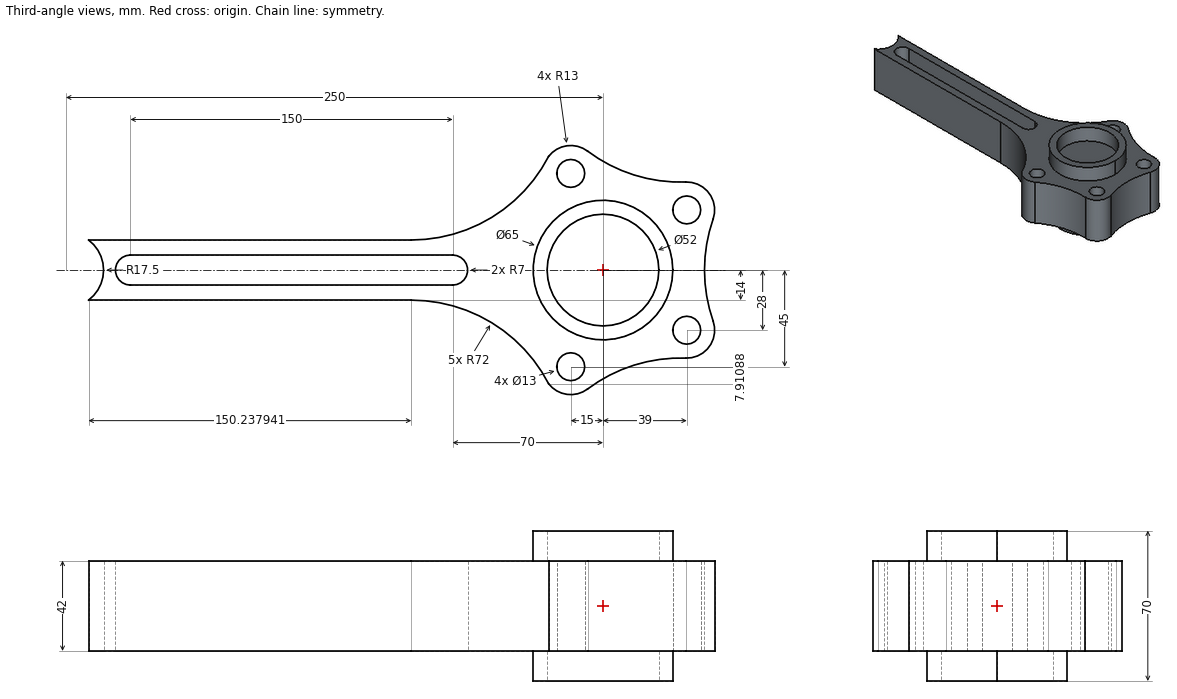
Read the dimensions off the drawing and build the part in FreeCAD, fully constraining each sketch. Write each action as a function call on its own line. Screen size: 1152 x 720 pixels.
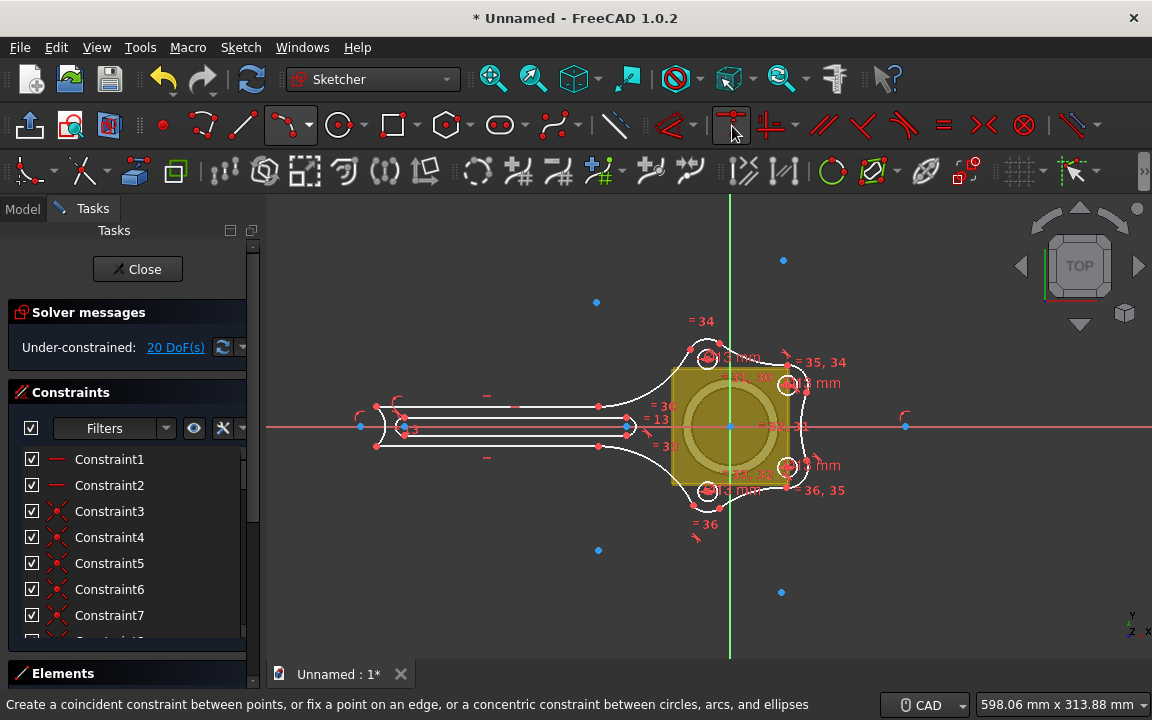
click(784, 261)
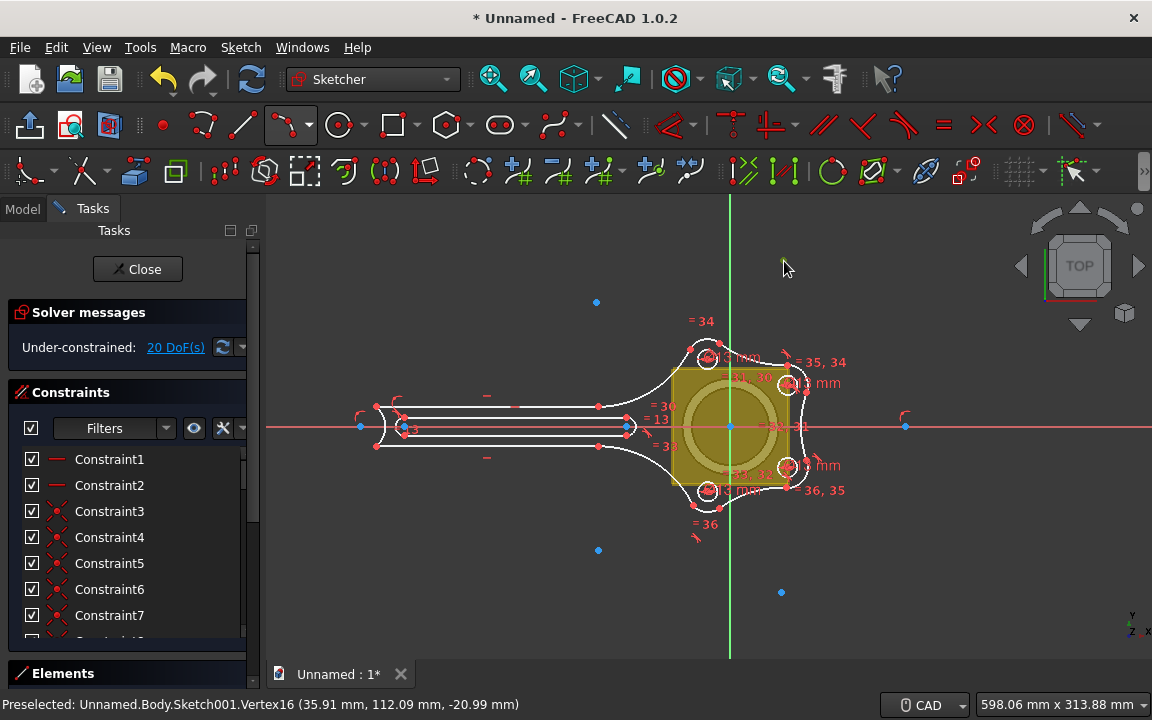
click(782, 592)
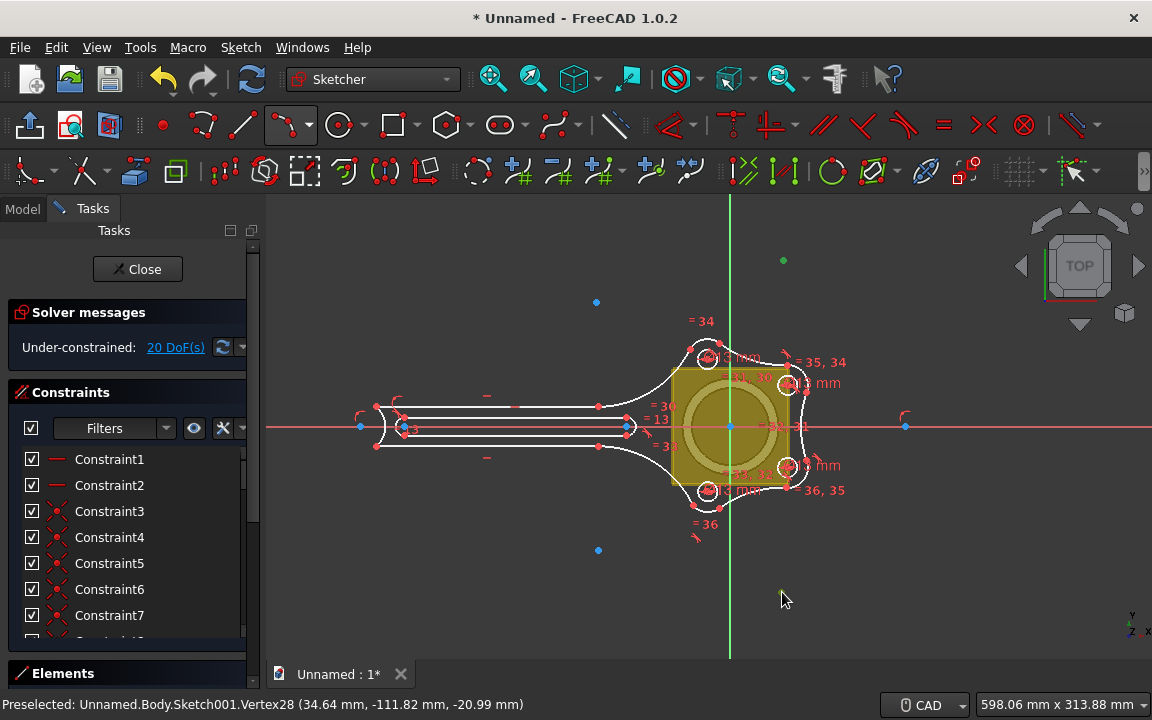
click(343, 427)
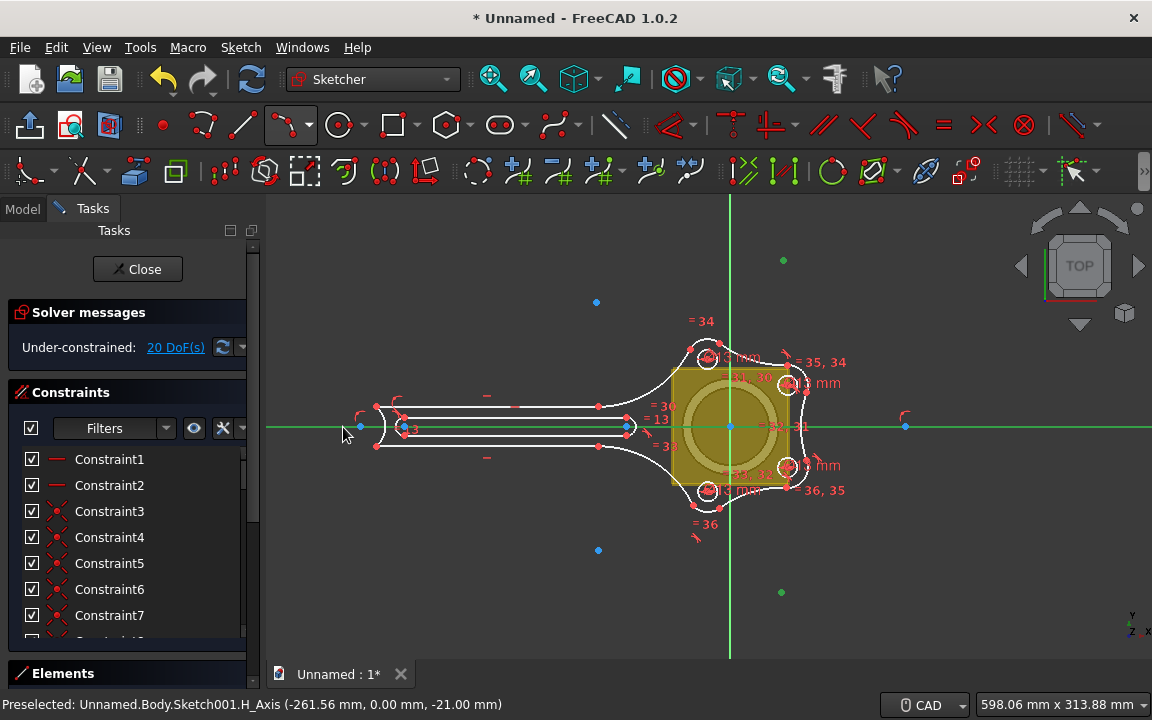
click(984, 126)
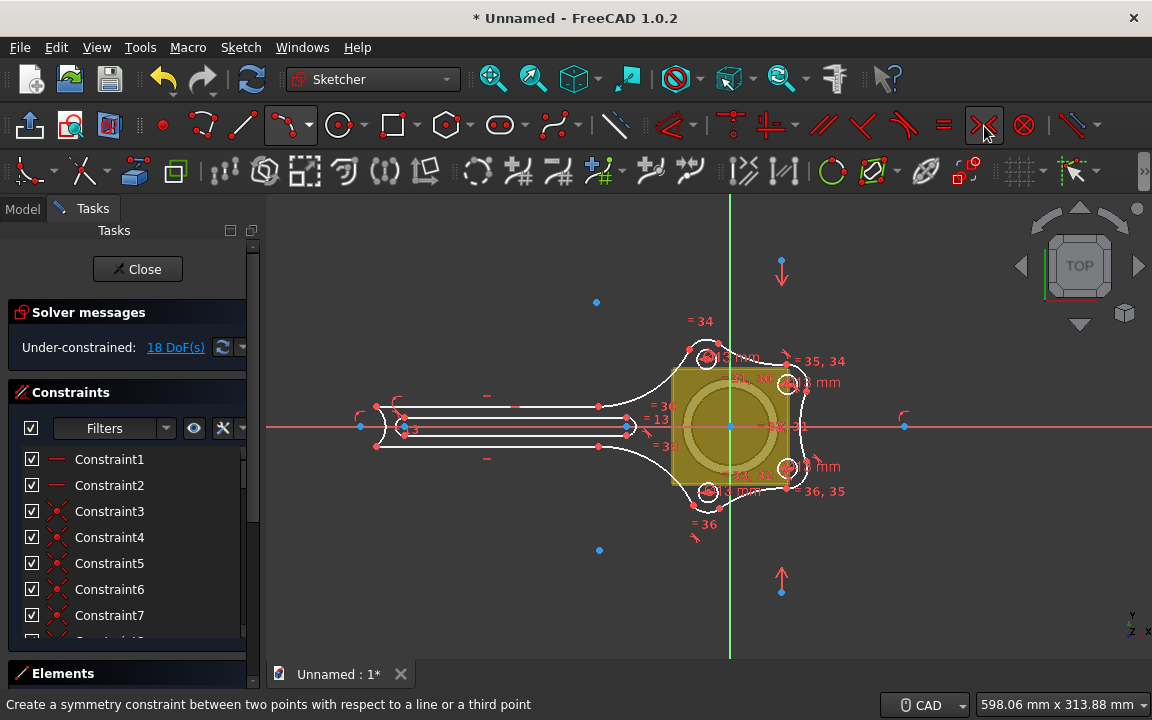
click(597, 302)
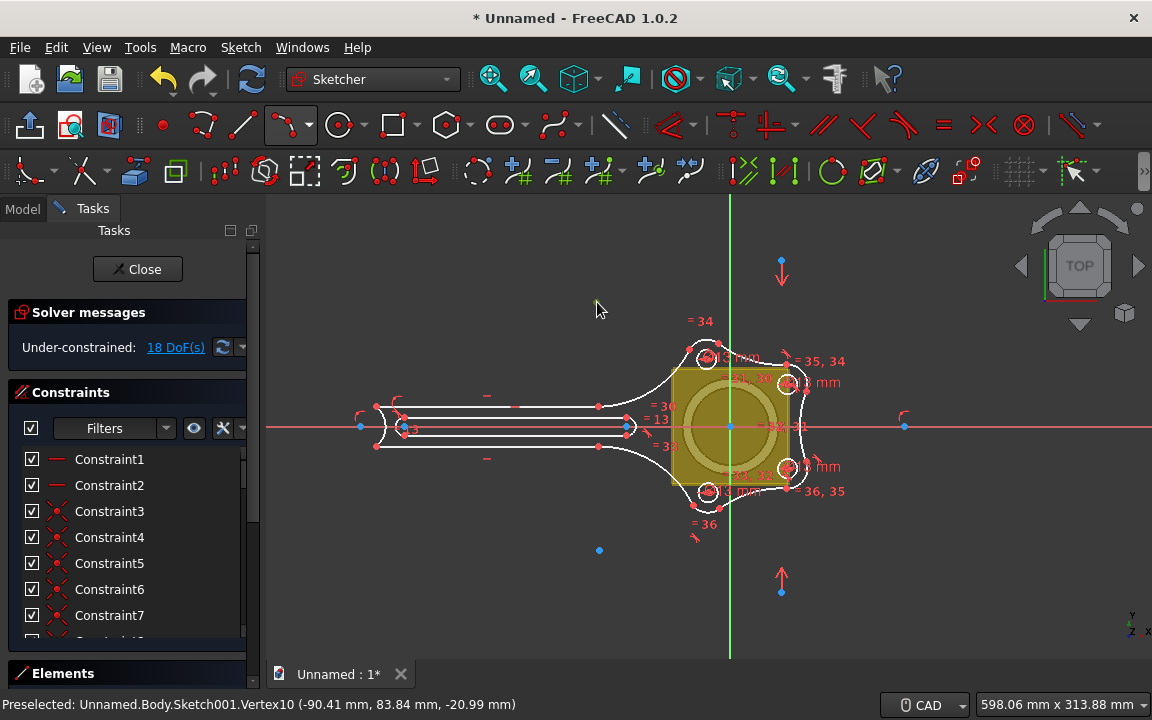
click(599, 551)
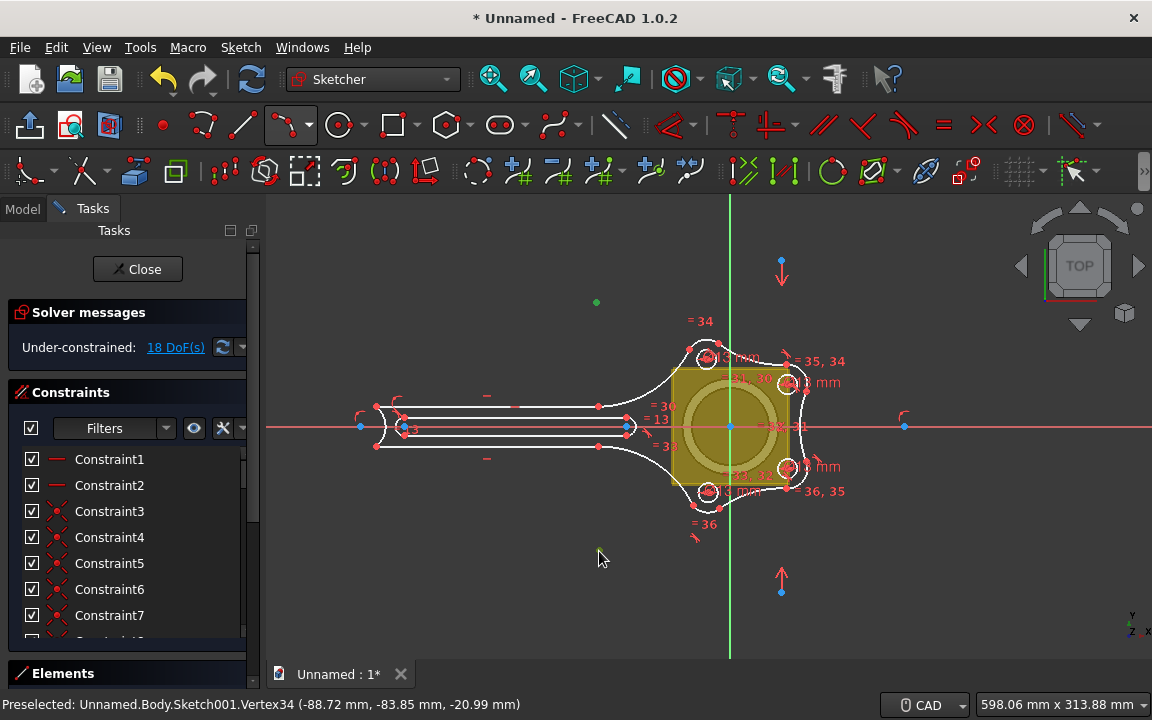
click(343, 427)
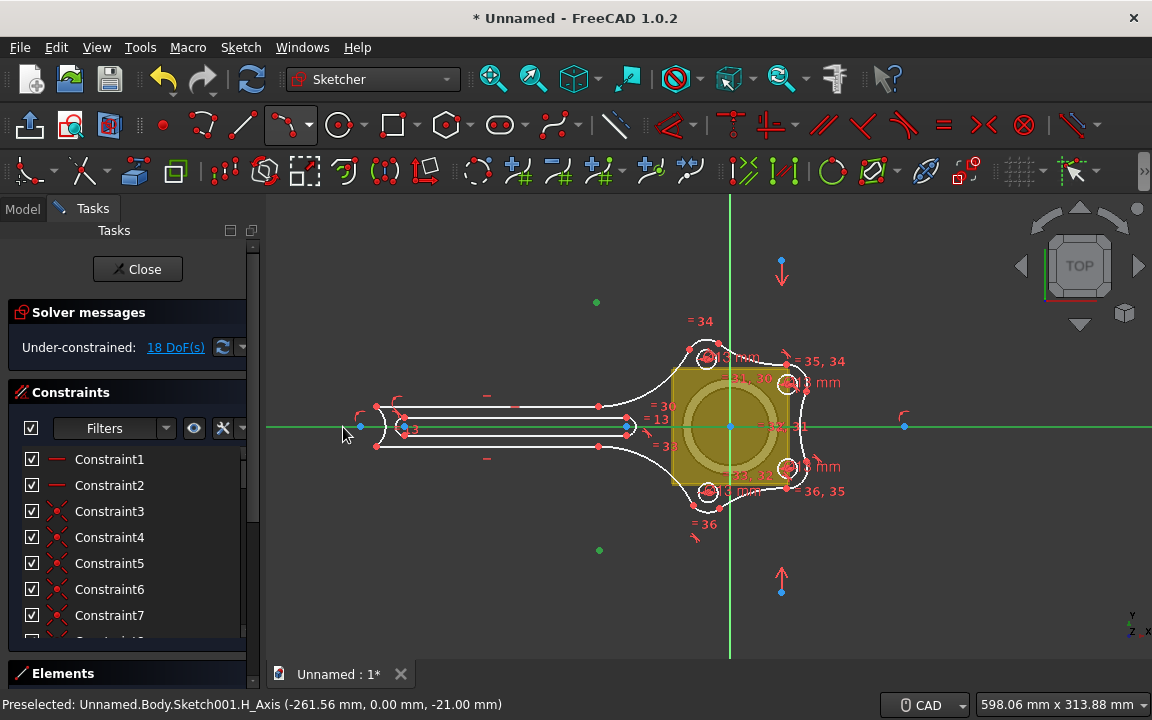
click(984, 126)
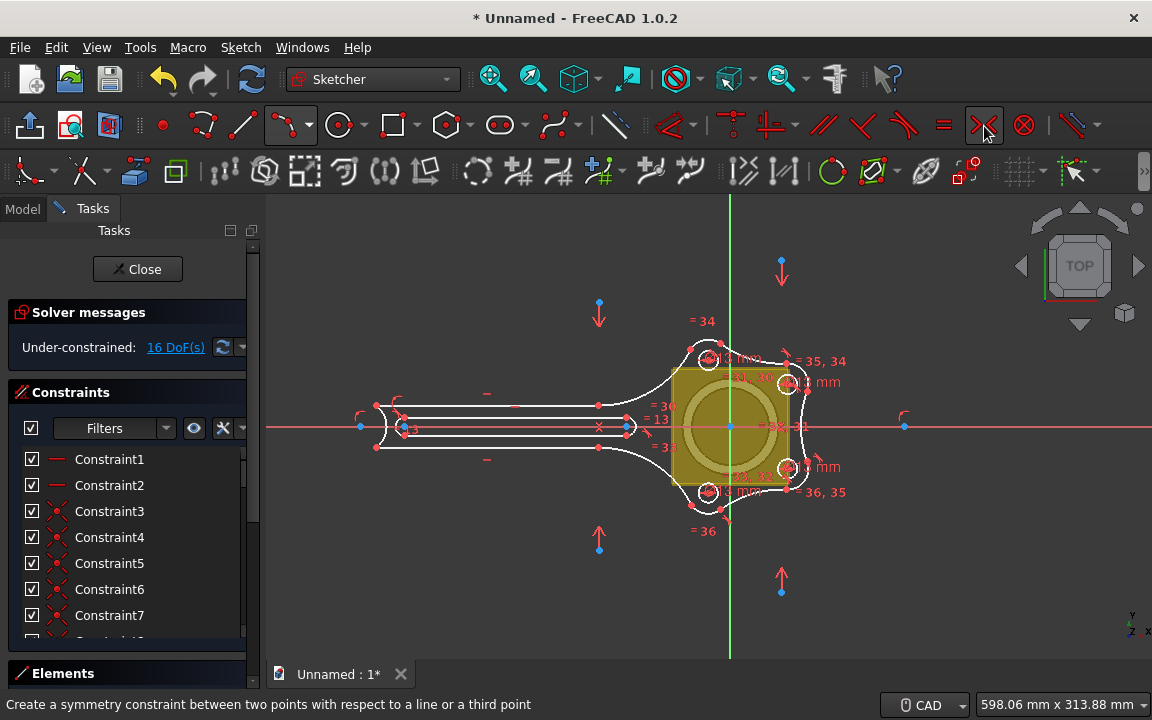
scroll(385, 436, up, 3)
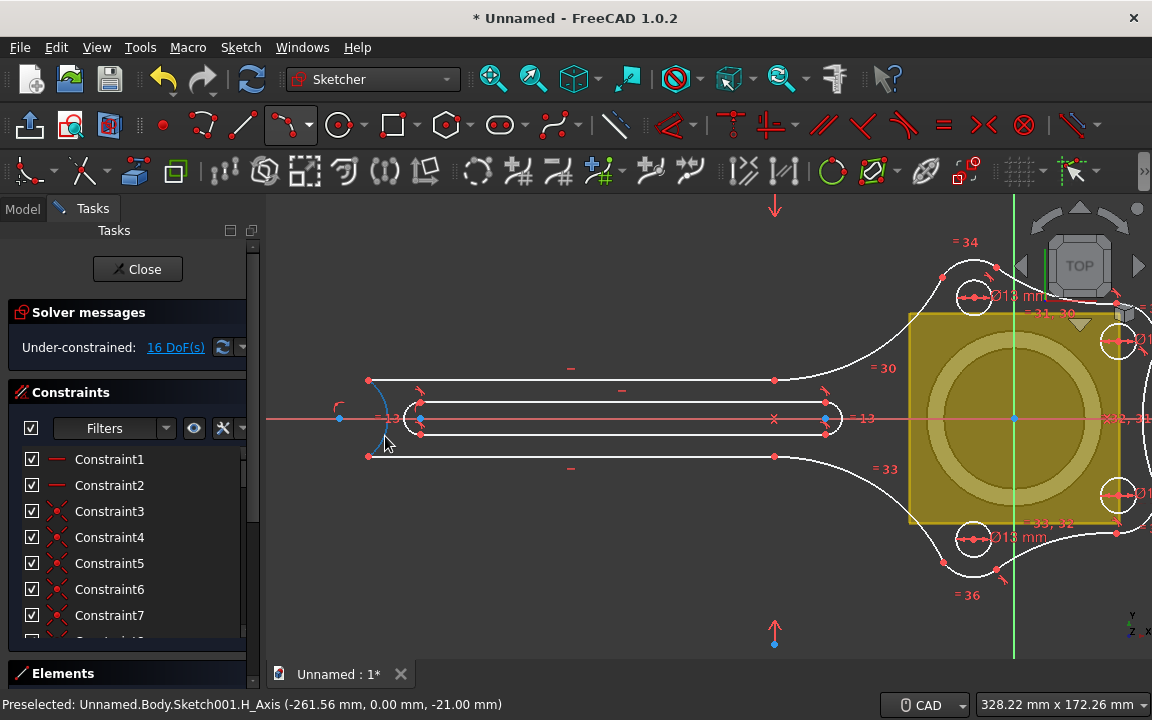
click(384, 436)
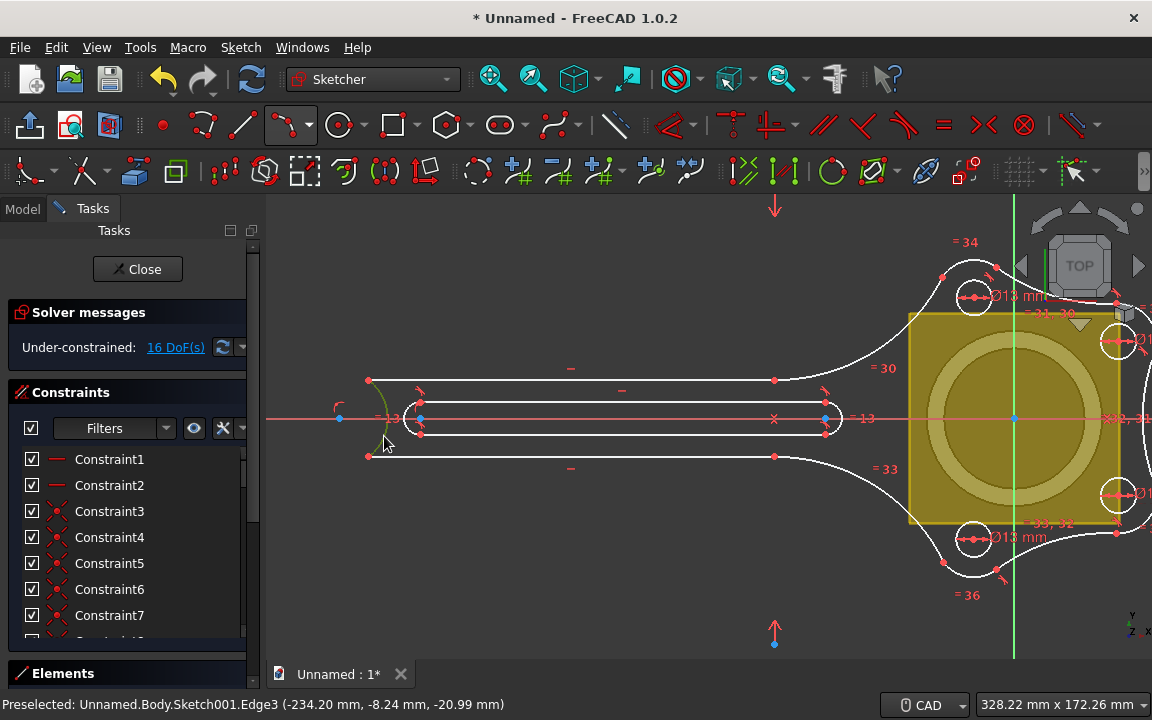
key(k)
key(r)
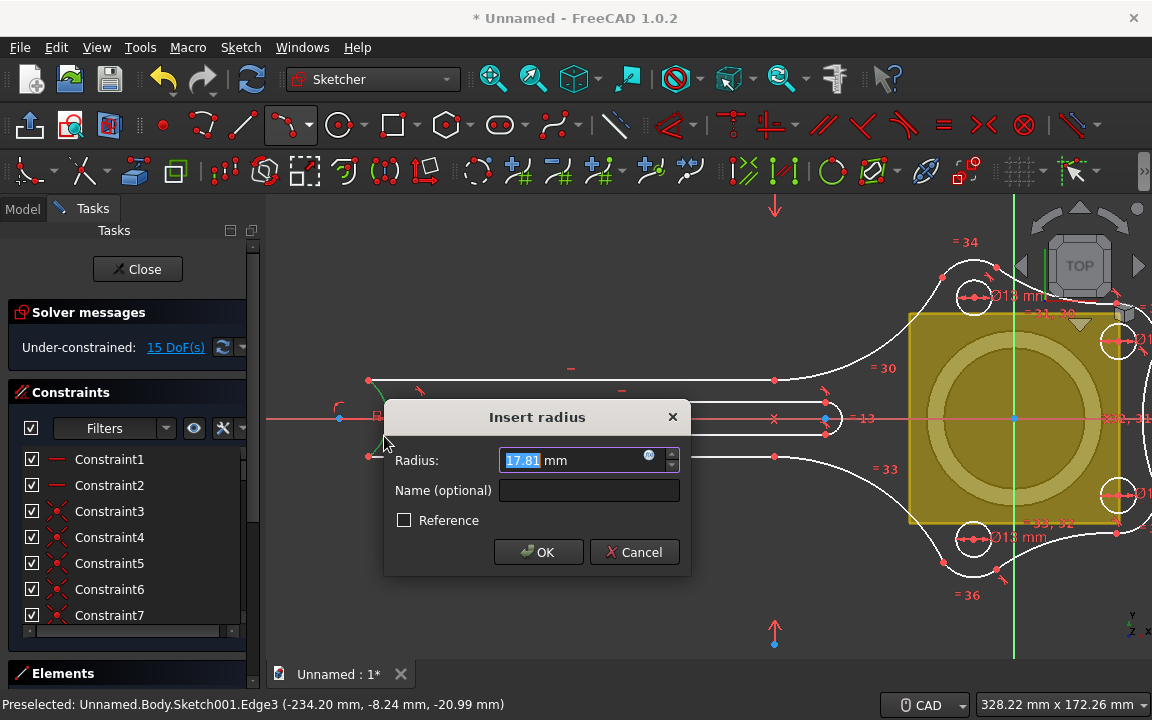
text(17.5)
key(Return)